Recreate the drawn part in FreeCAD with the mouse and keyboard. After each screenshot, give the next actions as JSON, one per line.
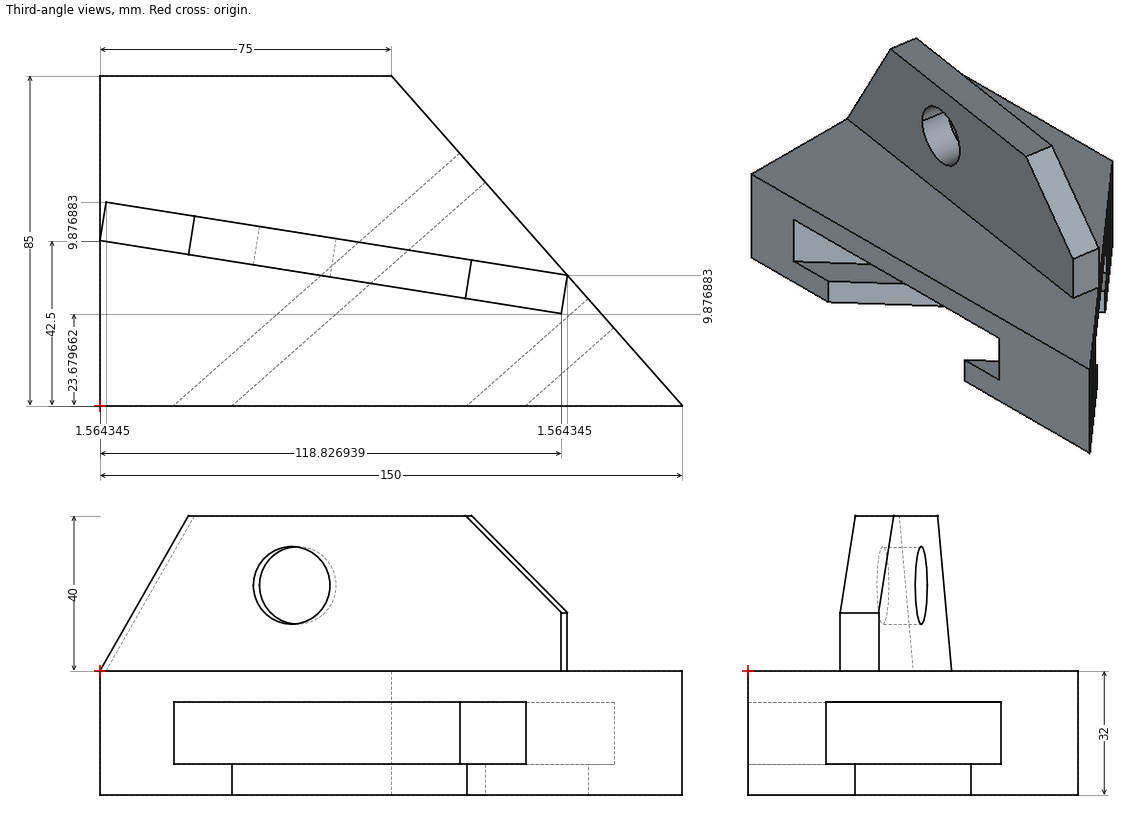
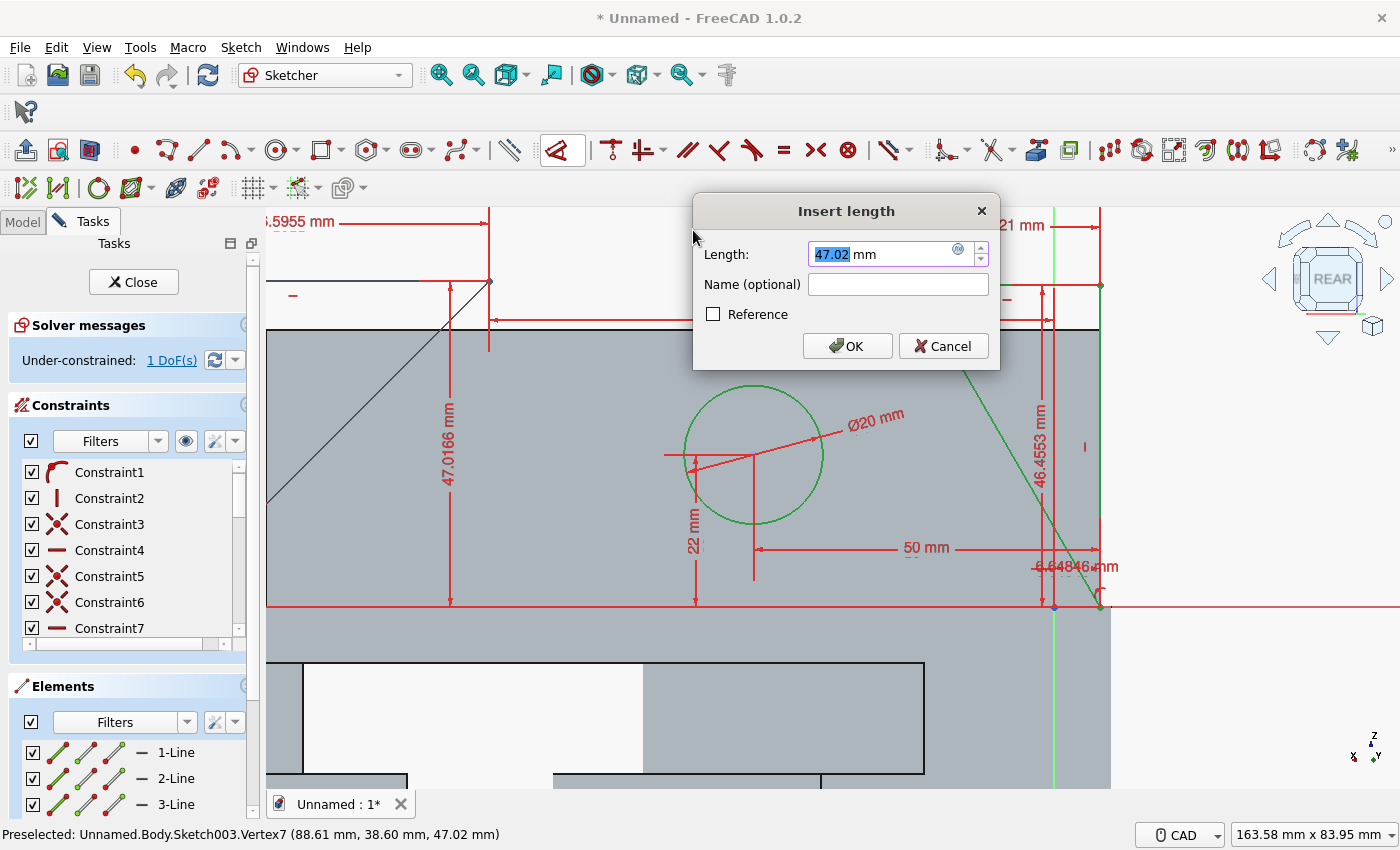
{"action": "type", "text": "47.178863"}
{"action": "key", "text": "Return"}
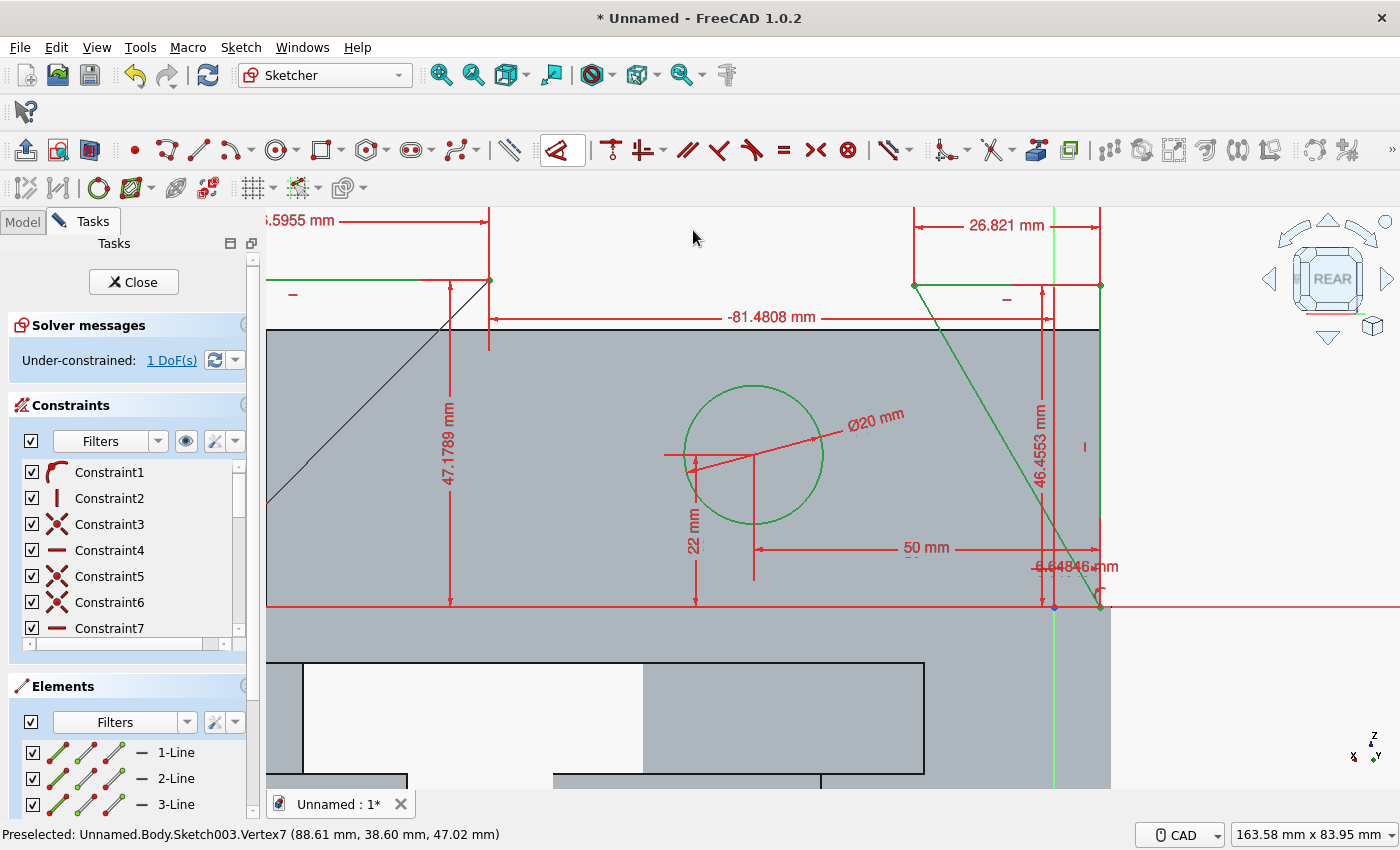
{"action": "scroll", "coordinate": [1102, 608], "scroll_direction": "down", "scroll_amount": 2}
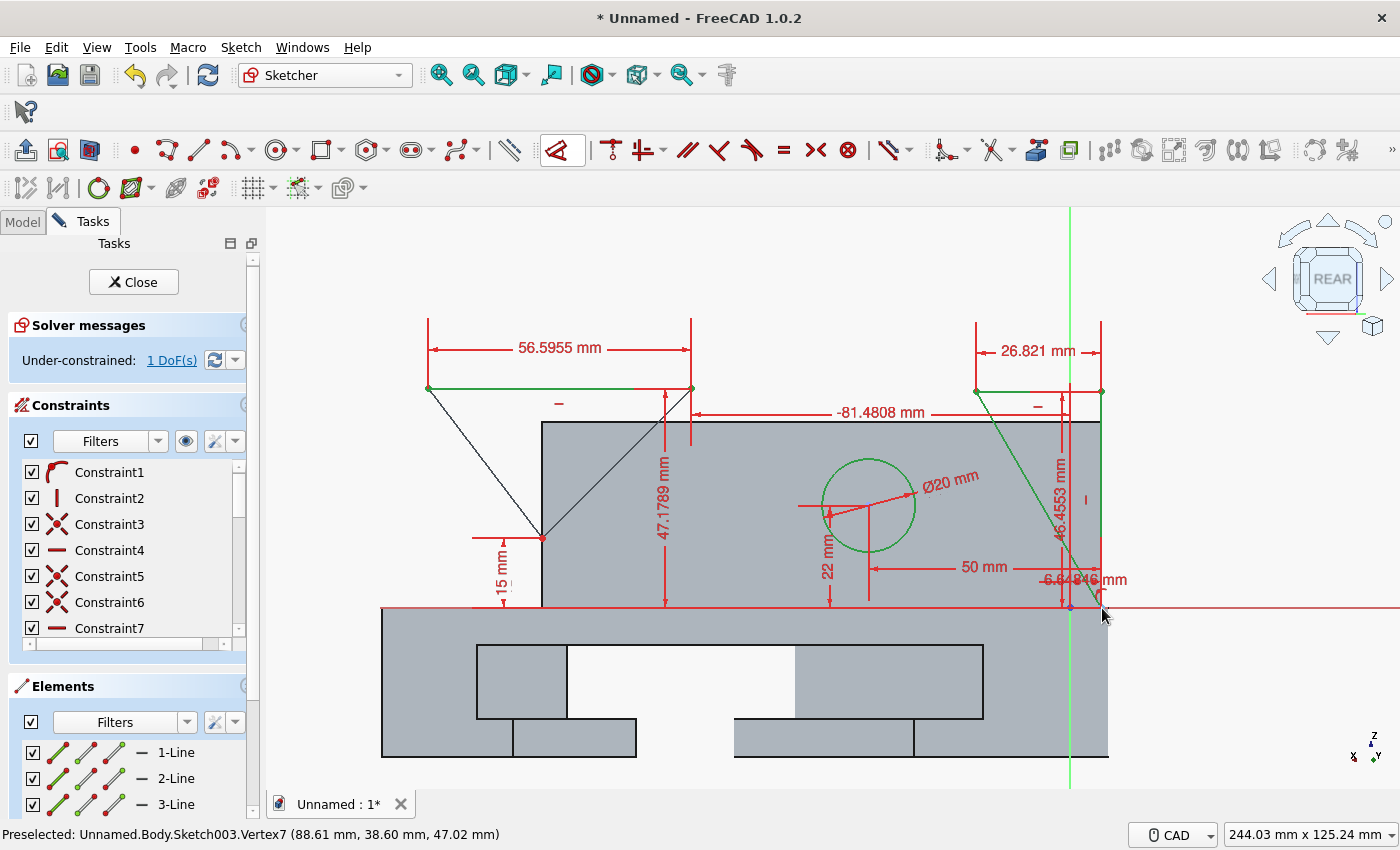
{"action": "left_click", "coordinate": [463, 433]}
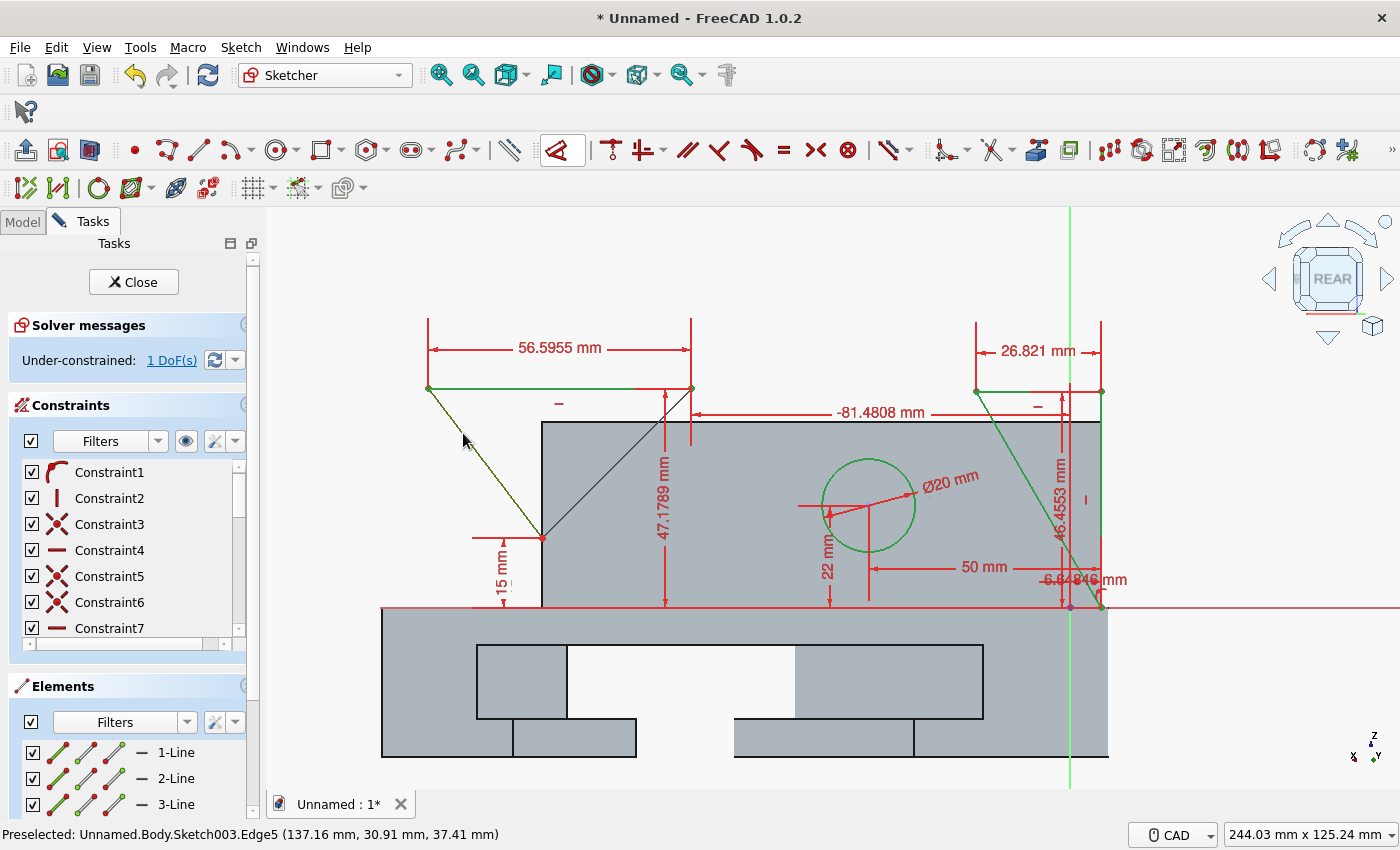
{"action": "key", "text": "l"}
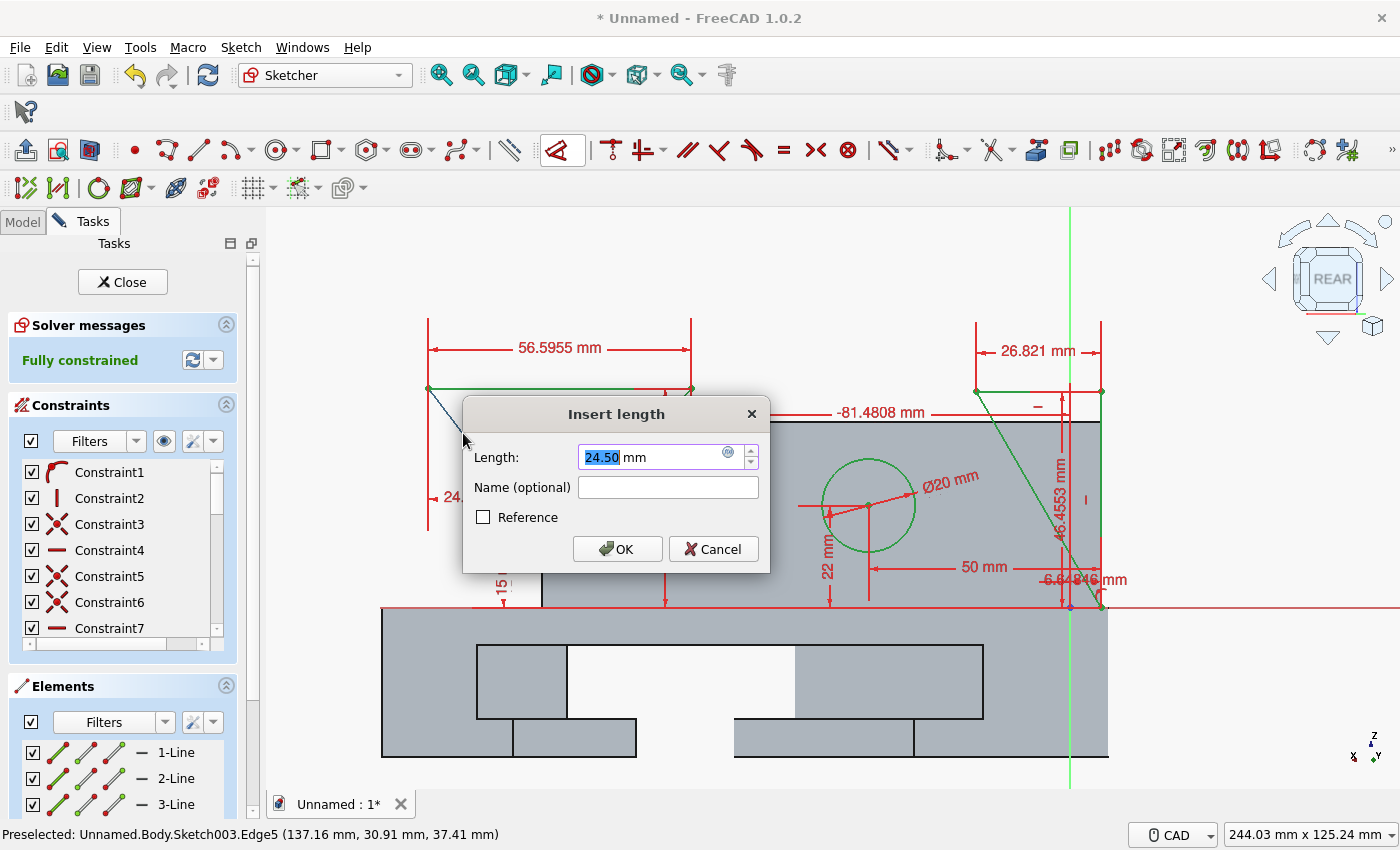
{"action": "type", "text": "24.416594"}
{"action": "key", "text": "Return"}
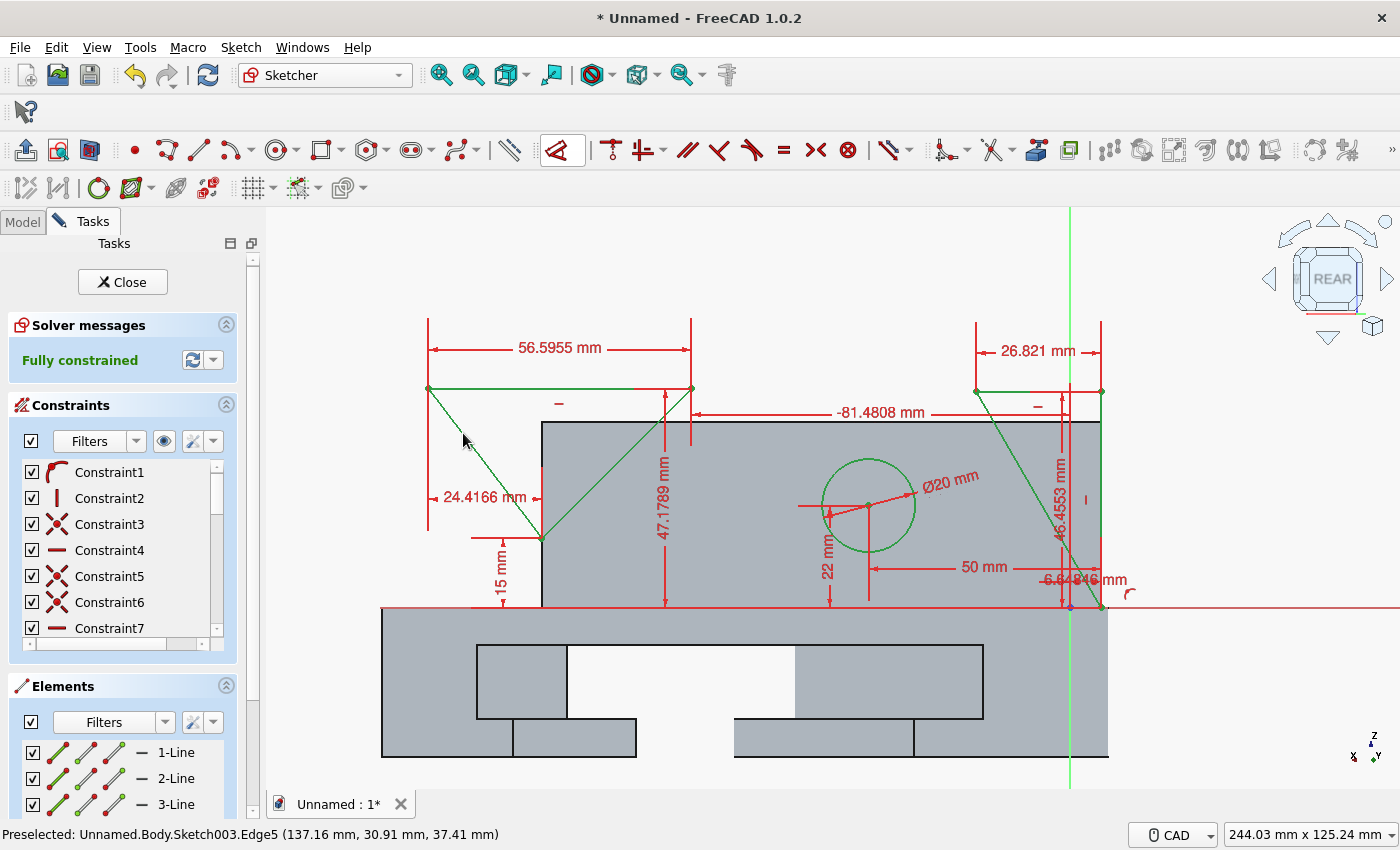
{"action": "left_click", "coordinate": [123, 282]}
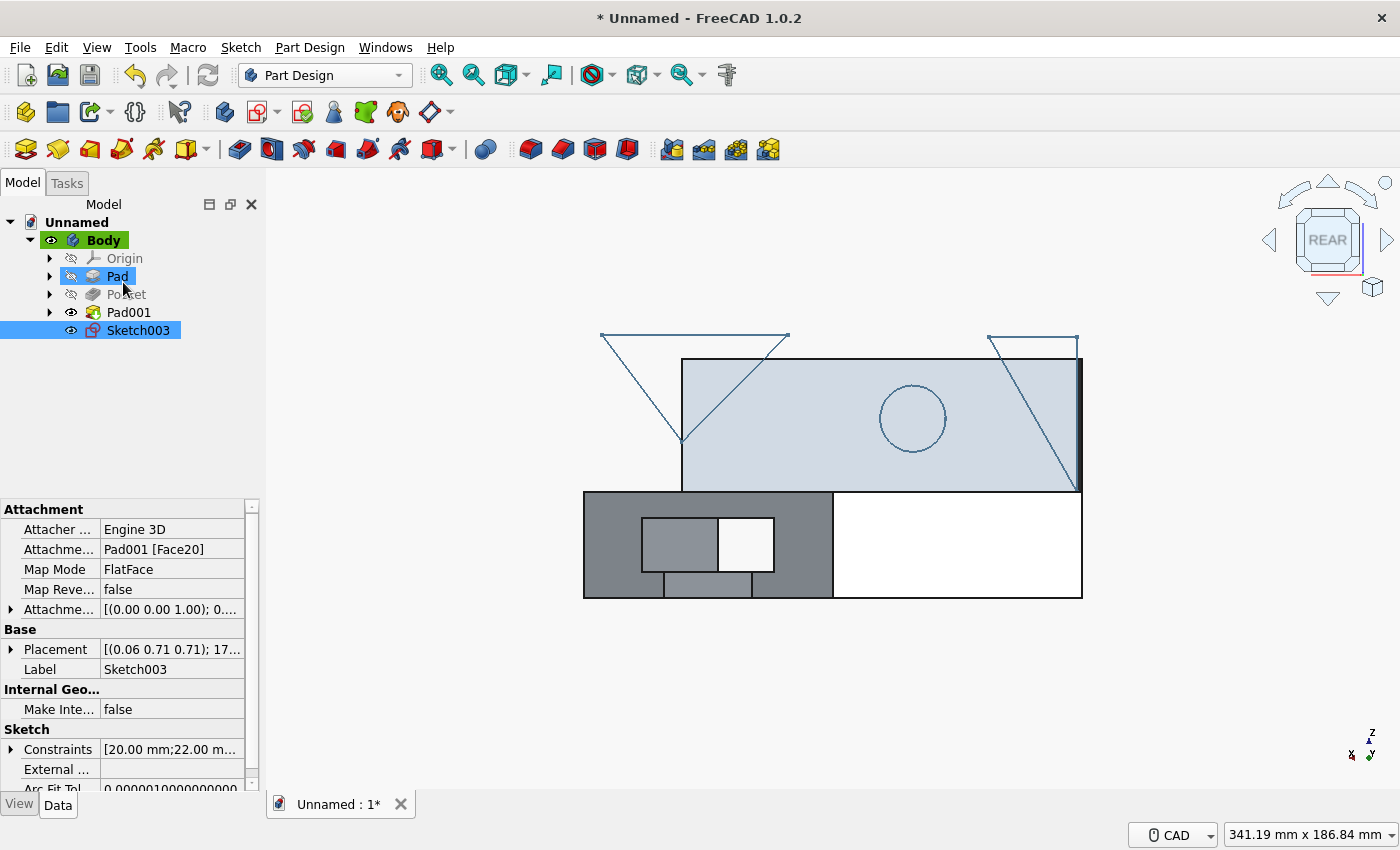
{"action": "left_click", "coordinate": [240, 150]}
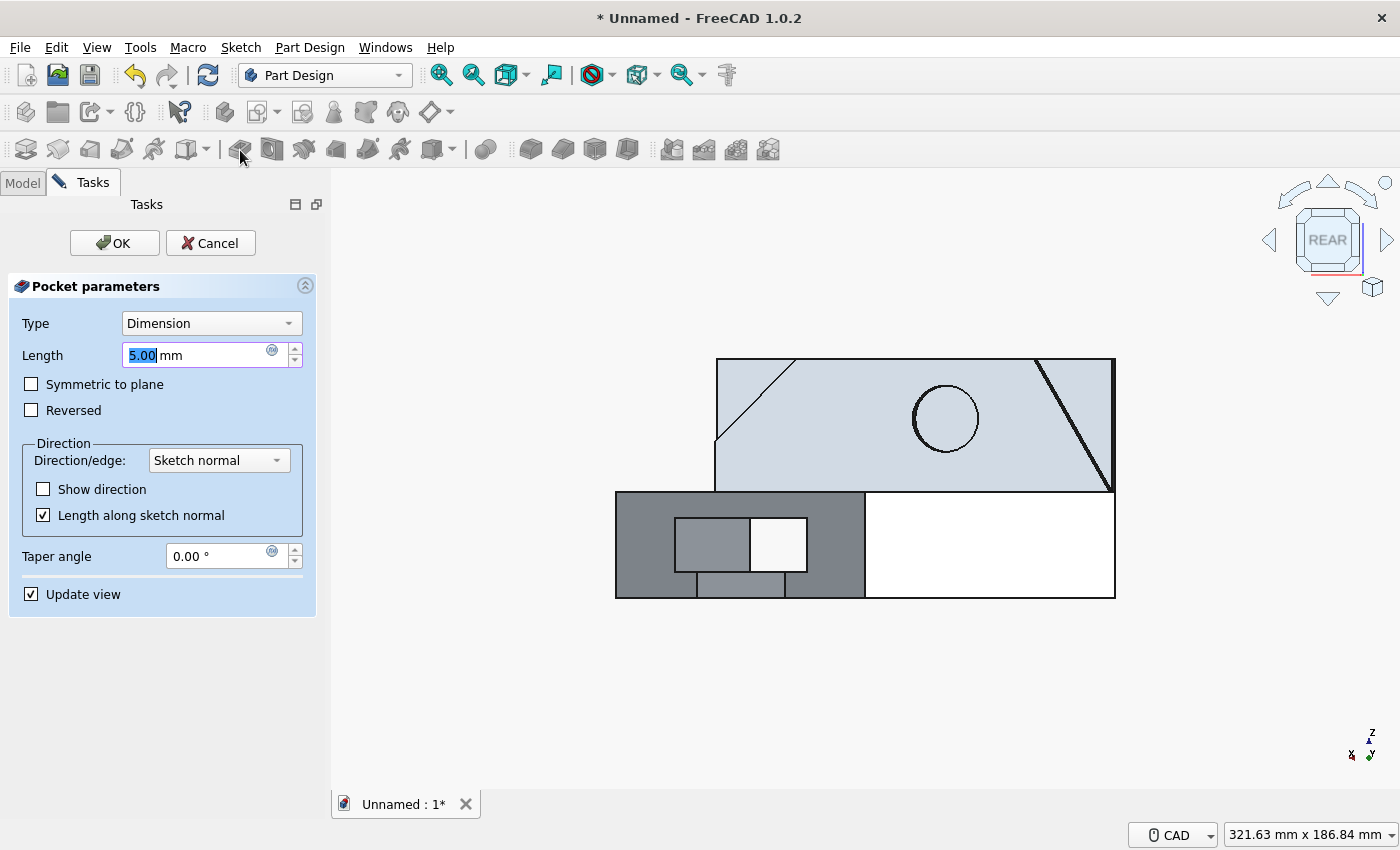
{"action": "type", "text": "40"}
{"action": "key", "text": "Tab"}